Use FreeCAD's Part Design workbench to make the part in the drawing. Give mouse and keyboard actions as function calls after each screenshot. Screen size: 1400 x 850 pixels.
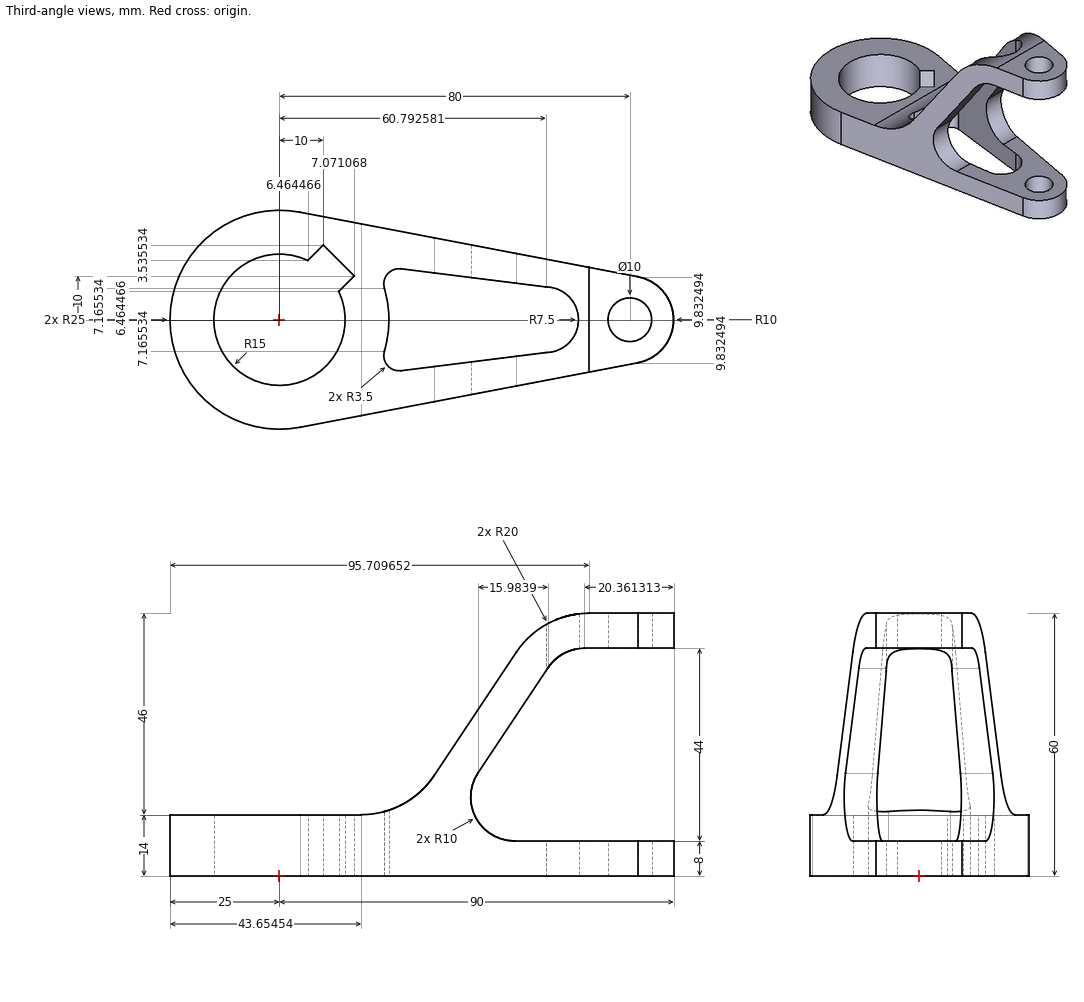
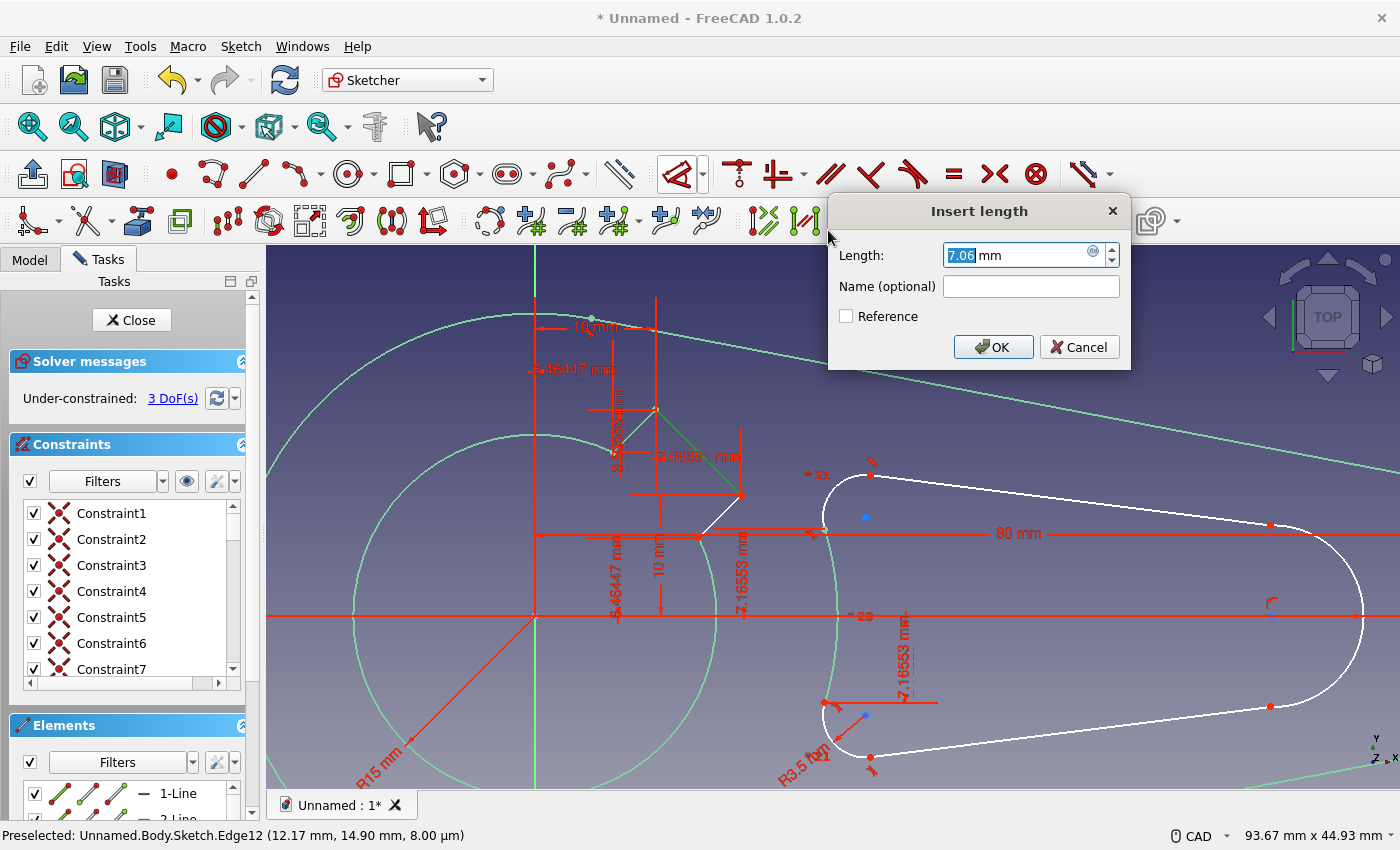
text(7.071068)
key(Return)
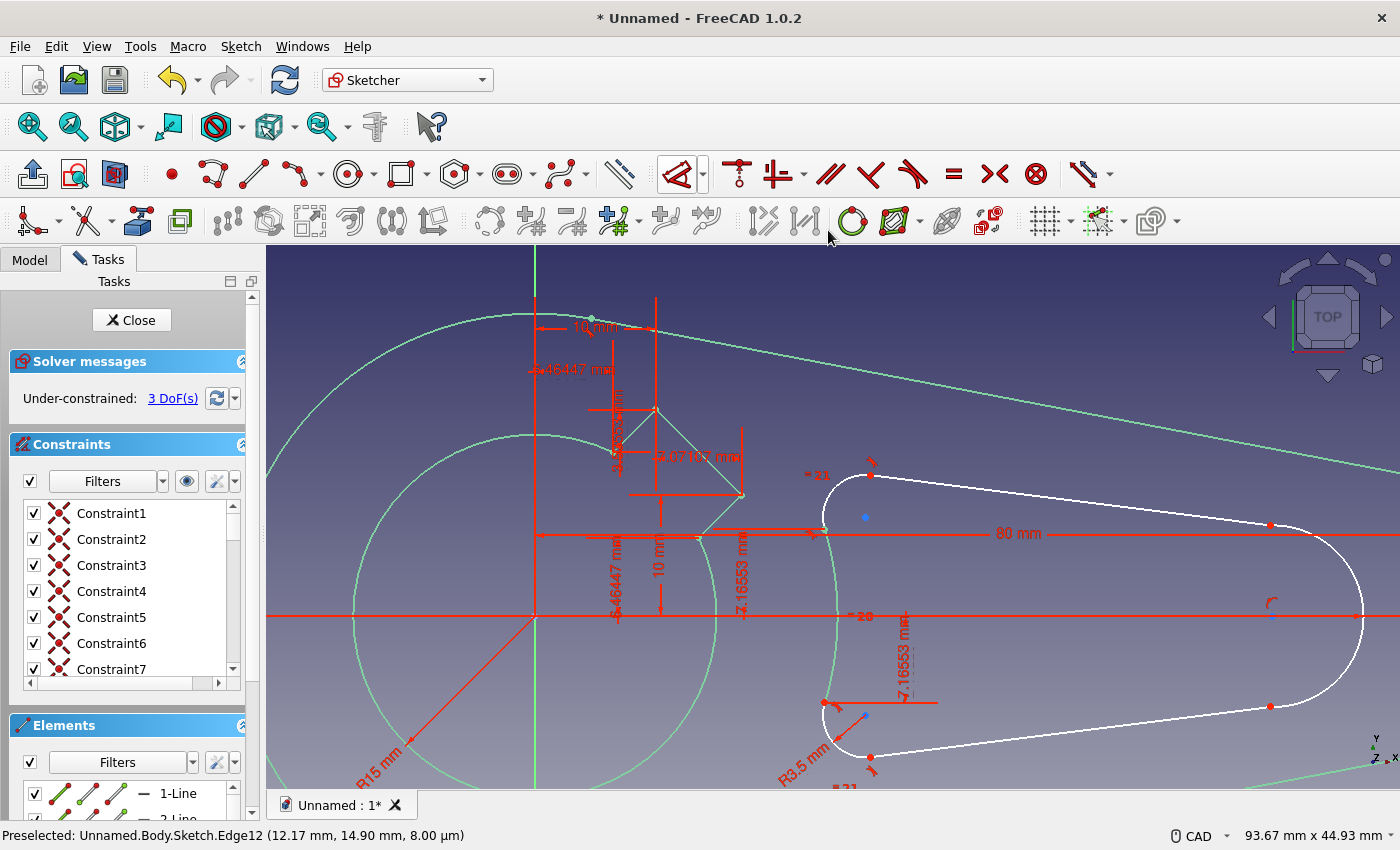
scroll(631, 436, down, 4)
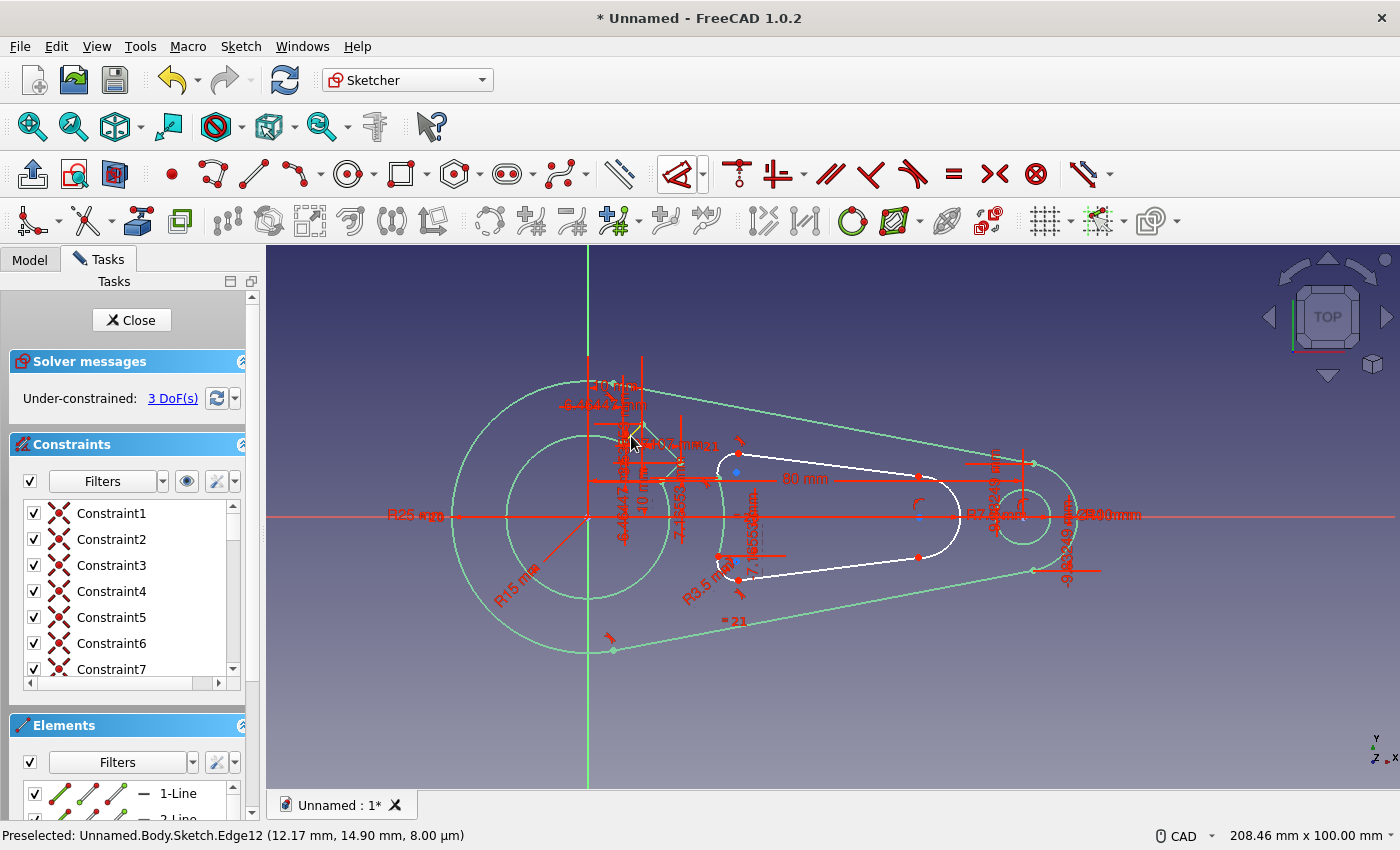
click(919, 476)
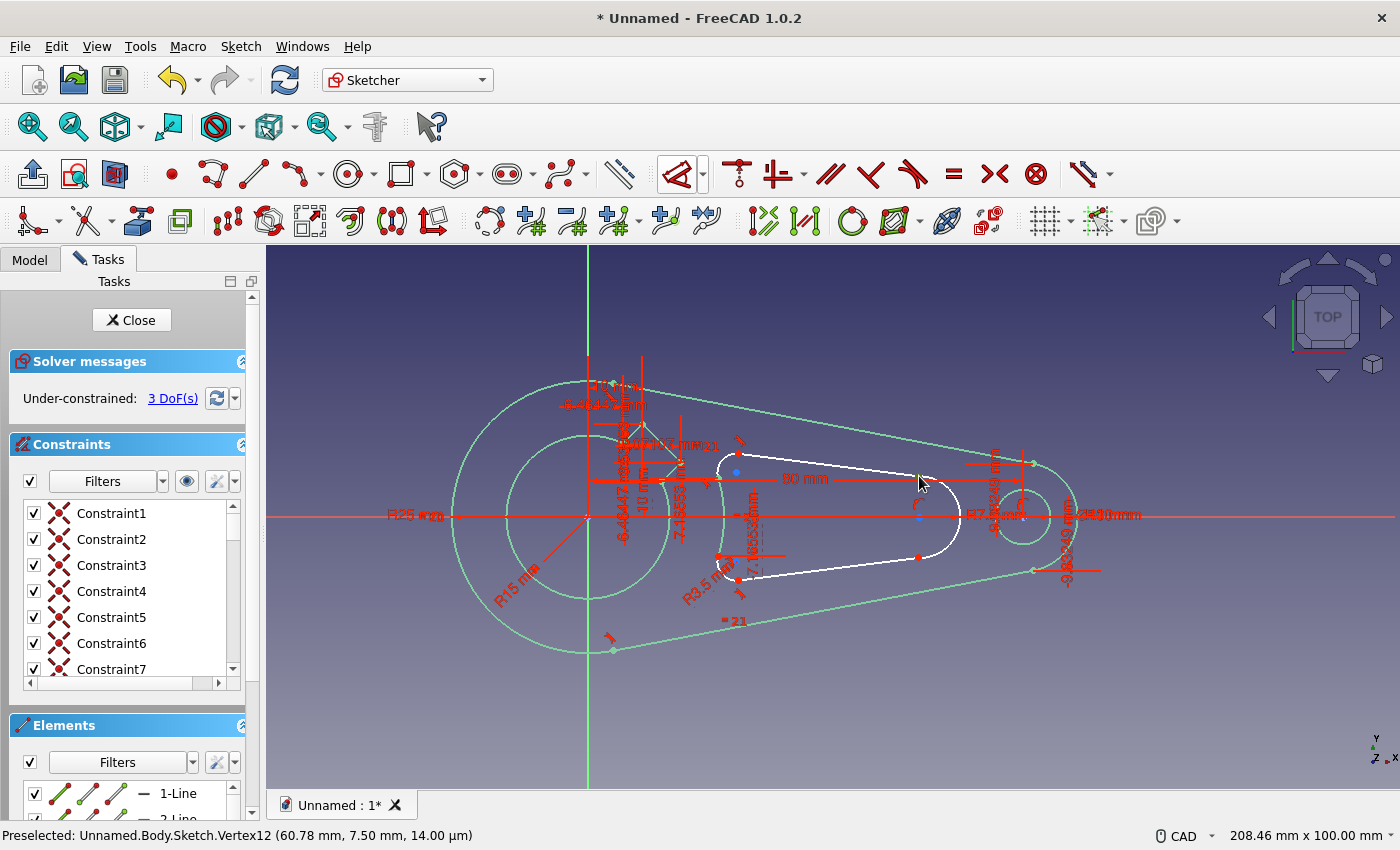
key(l)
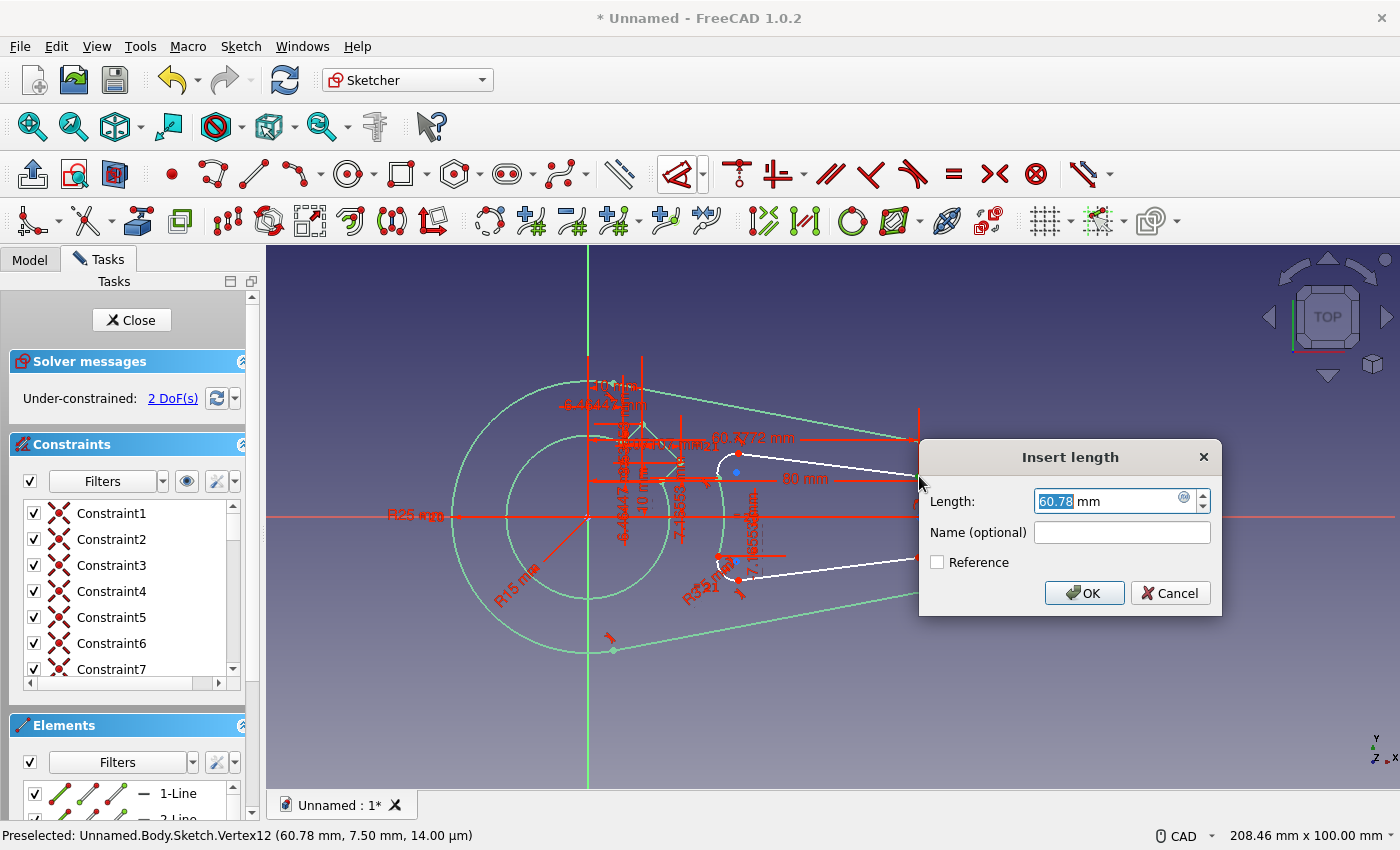
text(60.792581)
key(Return)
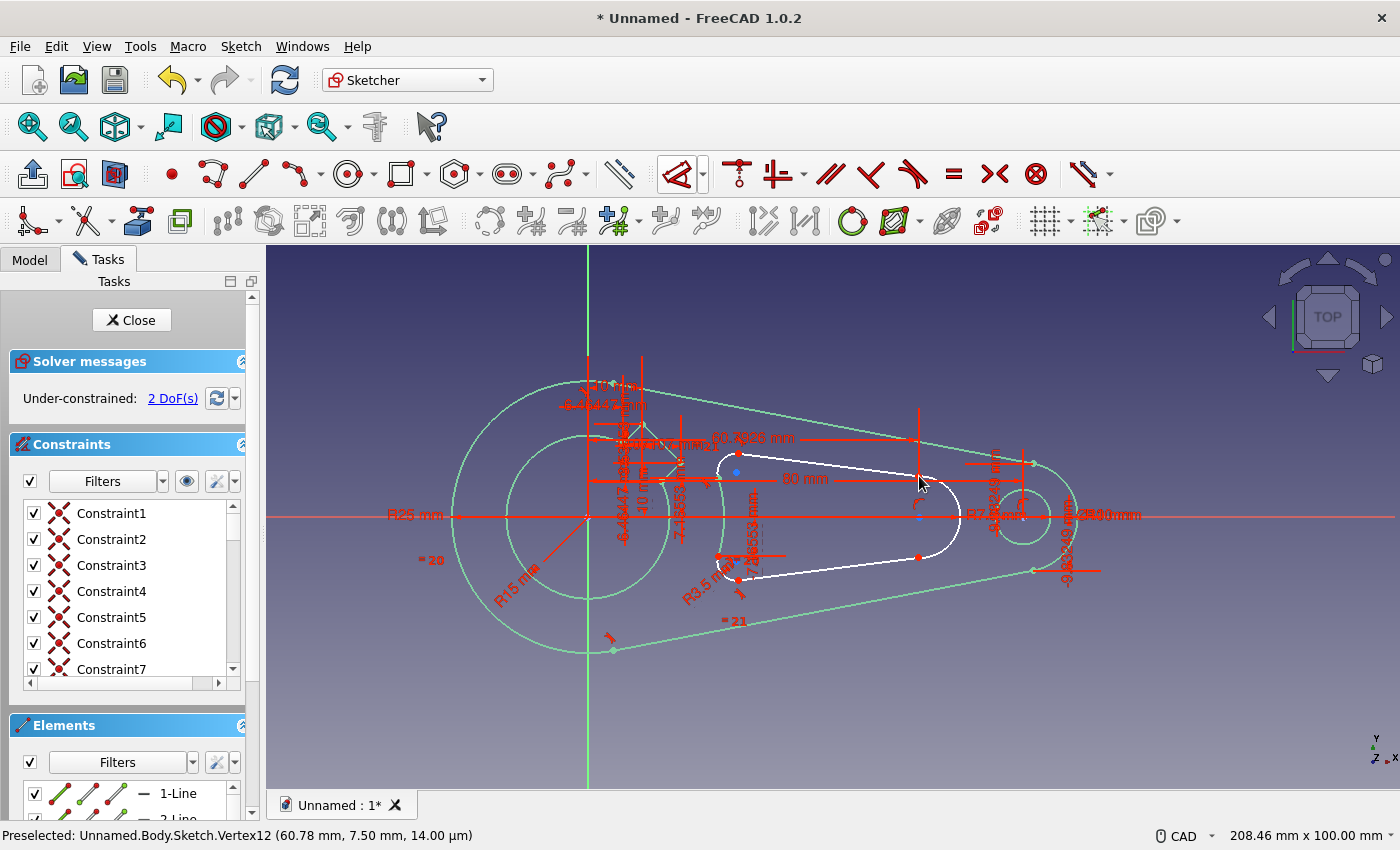
click(919, 558)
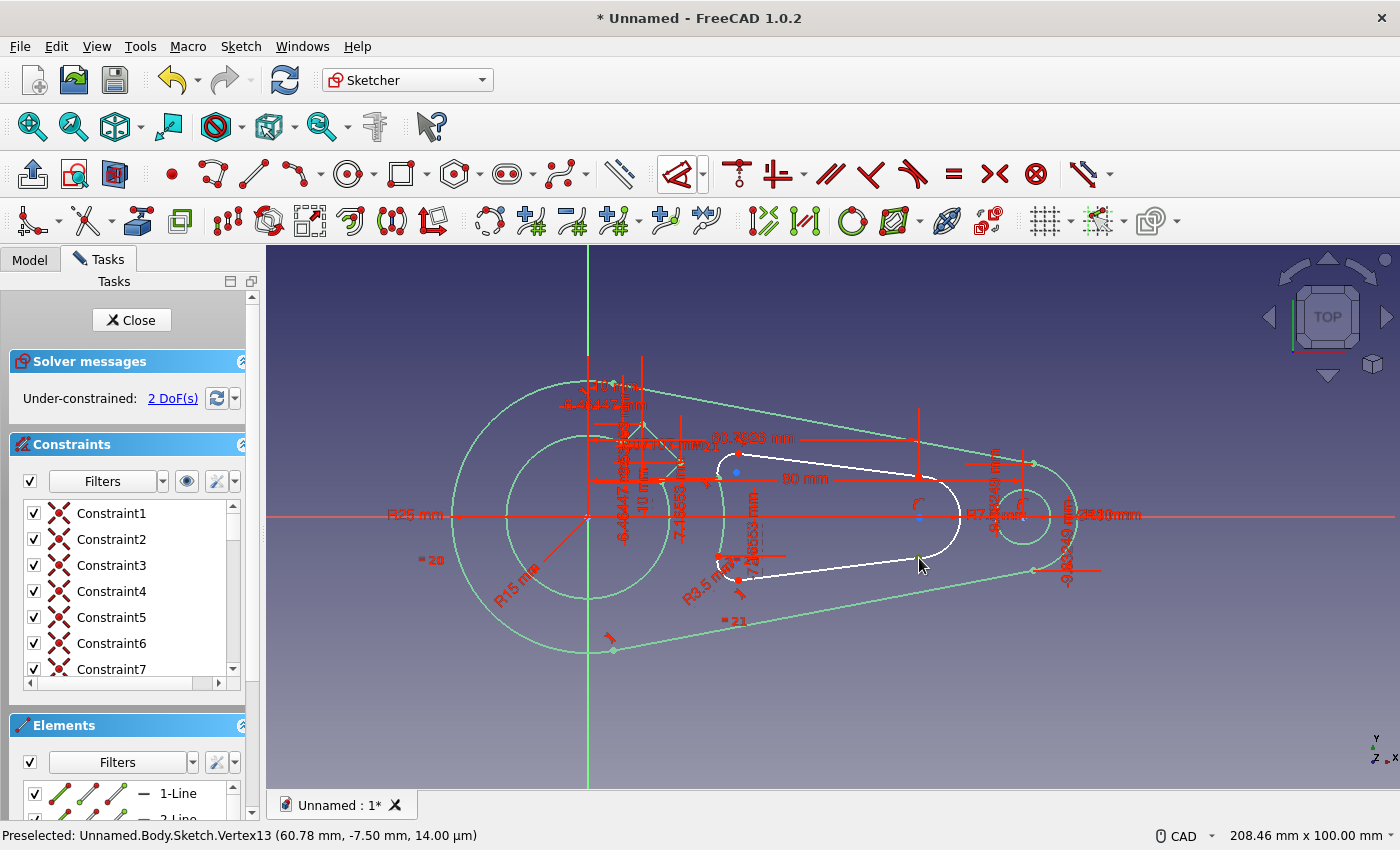
click(702, 174)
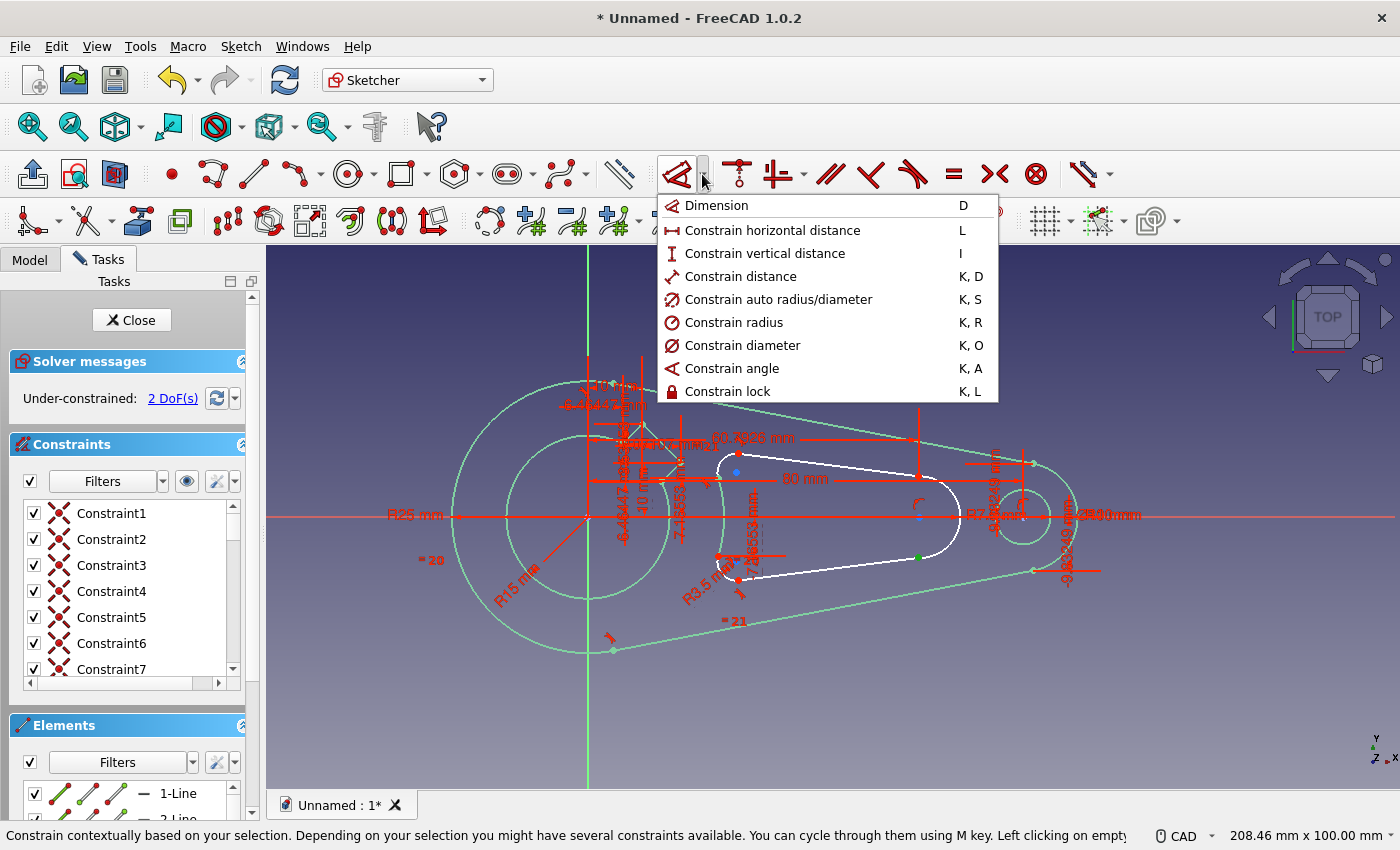
click(828, 230)